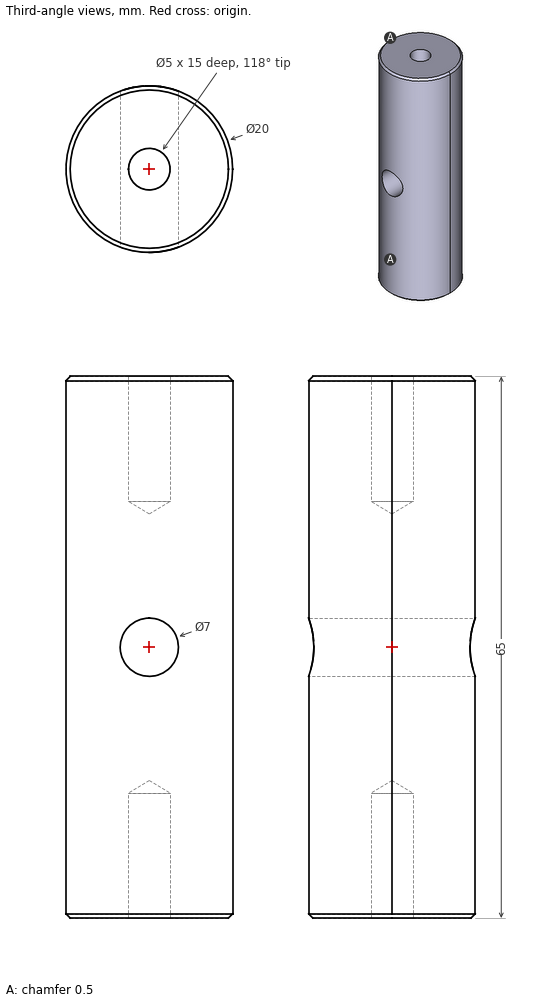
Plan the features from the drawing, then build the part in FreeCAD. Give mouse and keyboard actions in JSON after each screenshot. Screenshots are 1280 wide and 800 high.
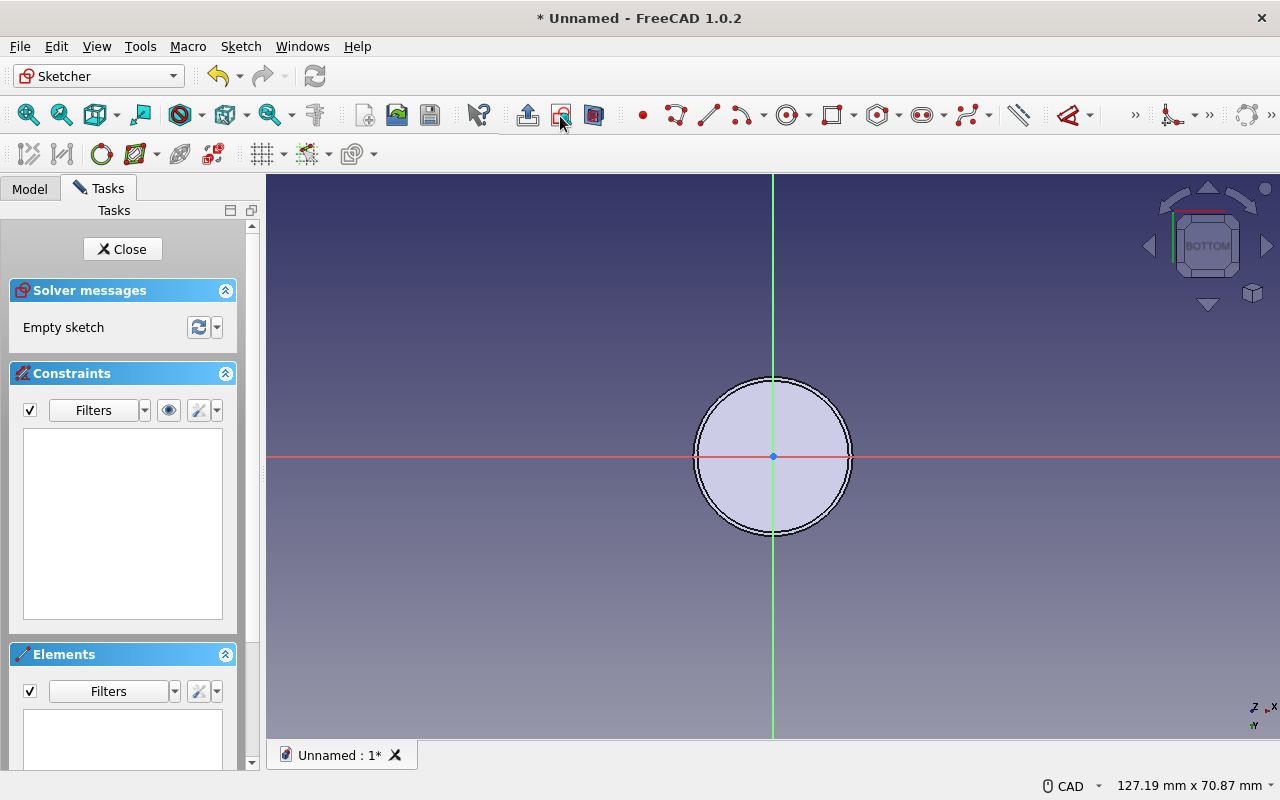
{"action": "scroll", "coordinate": [782, 456], "scroll_direction": "up", "scroll_amount": 11}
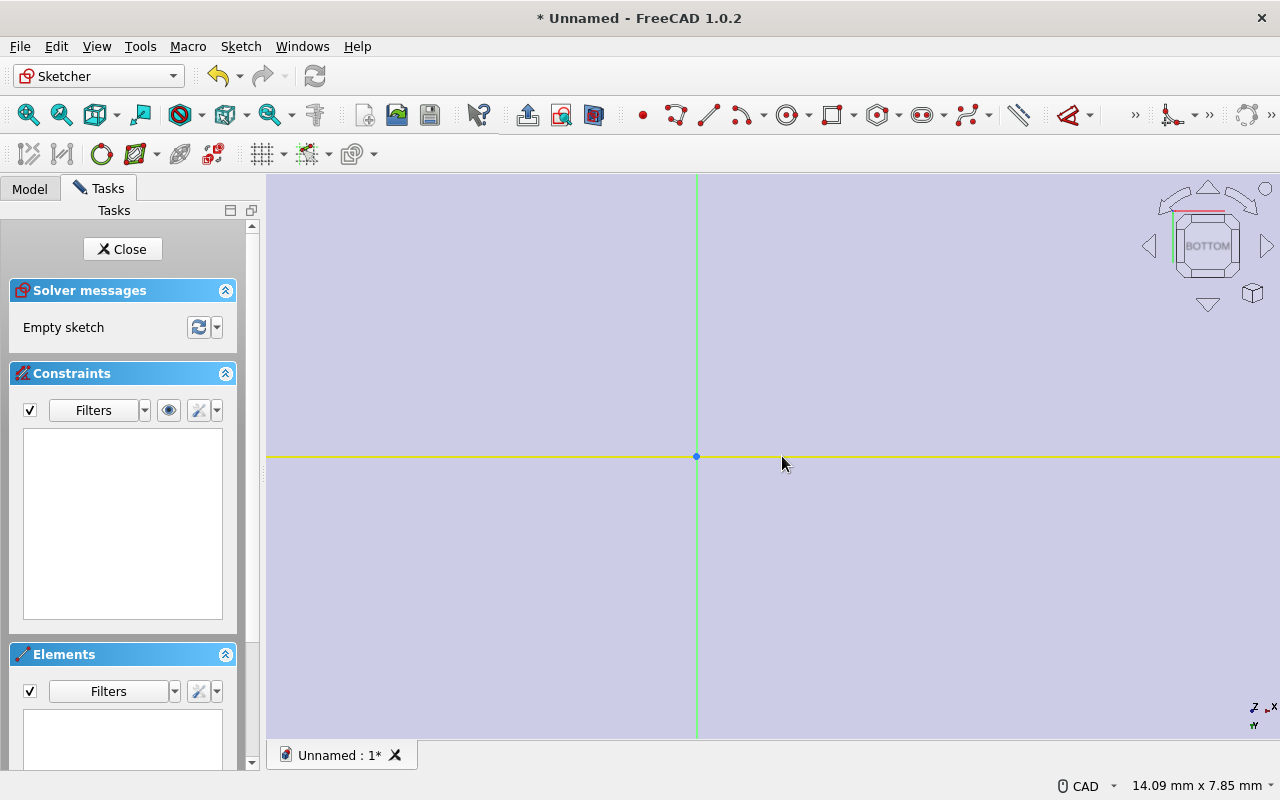
{"action": "left_click", "coordinate": [786, 116]}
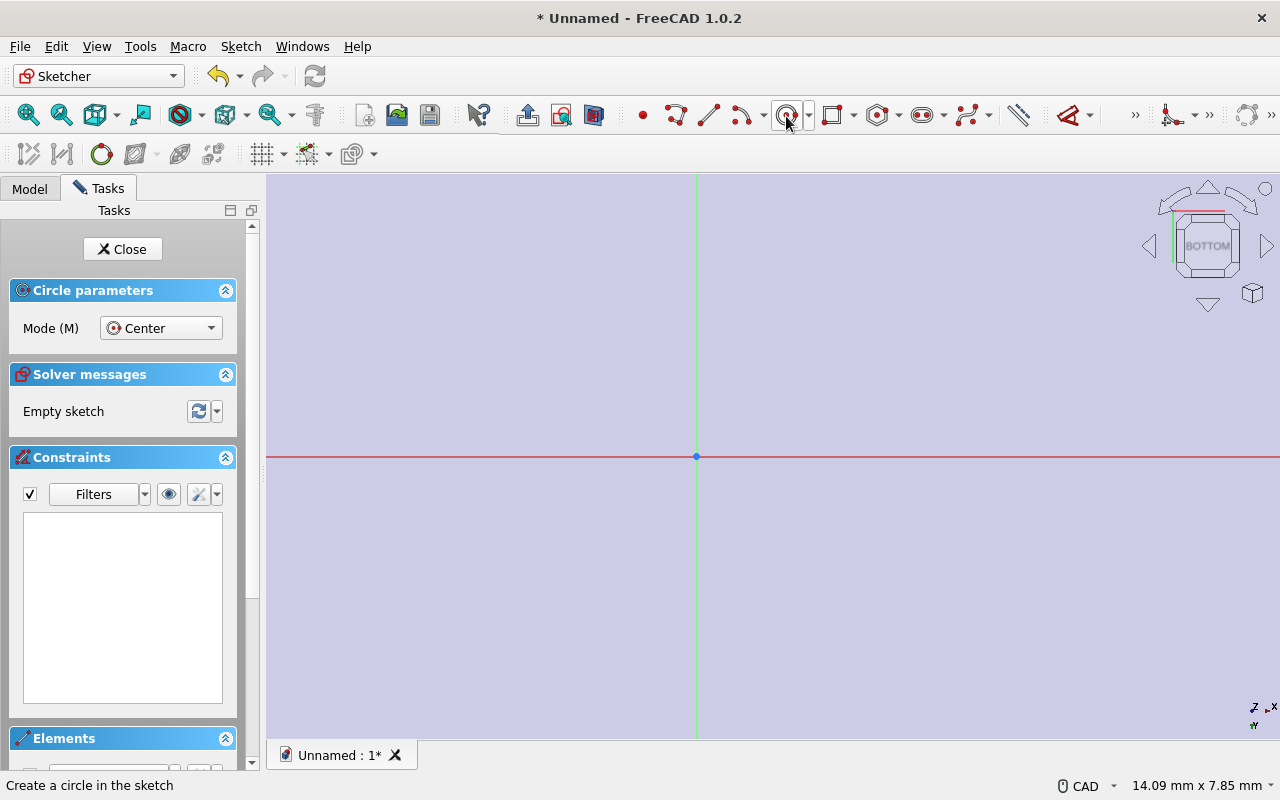
{"action": "left_click", "coordinate": [697, 456]}
{"action": "left_click", "coordinate": [824, 329]}
{"action": "key", "text": "Escape"}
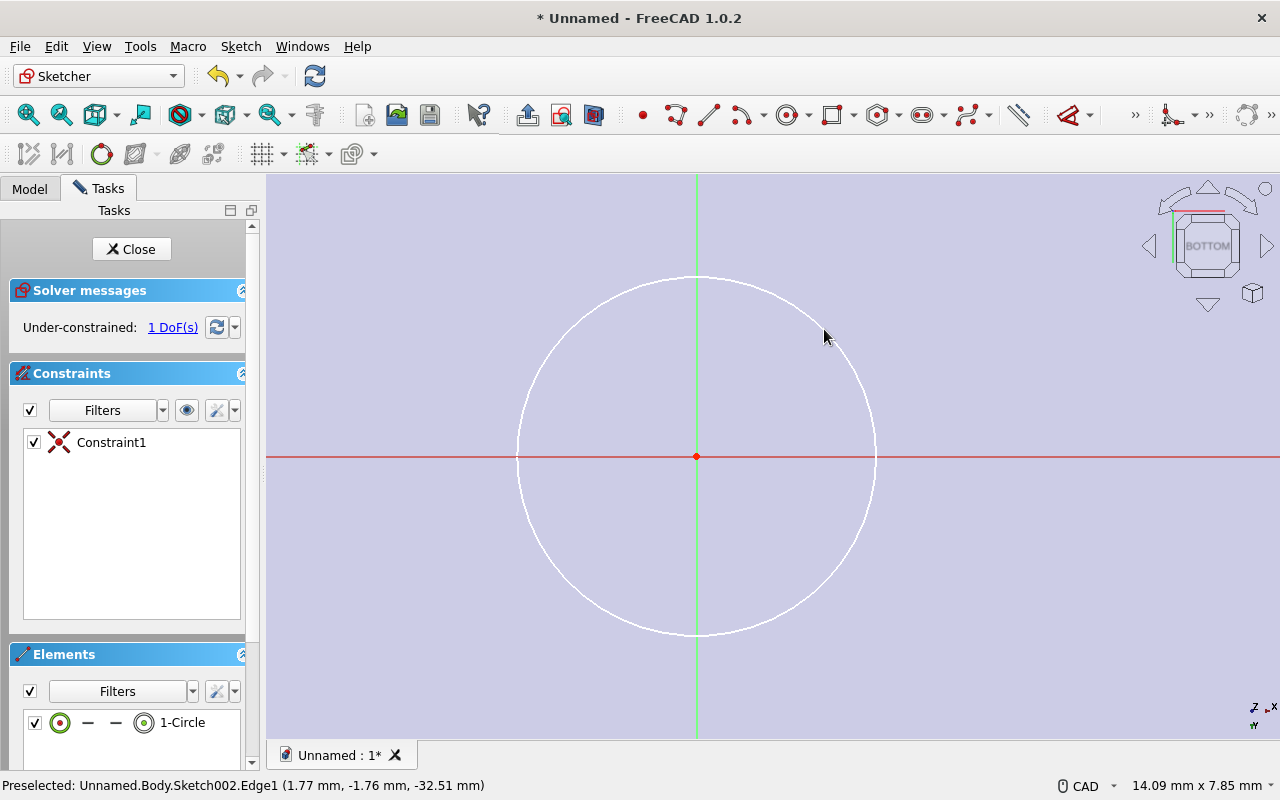
{"action": "left_click", "coordinate": [1068, 116]}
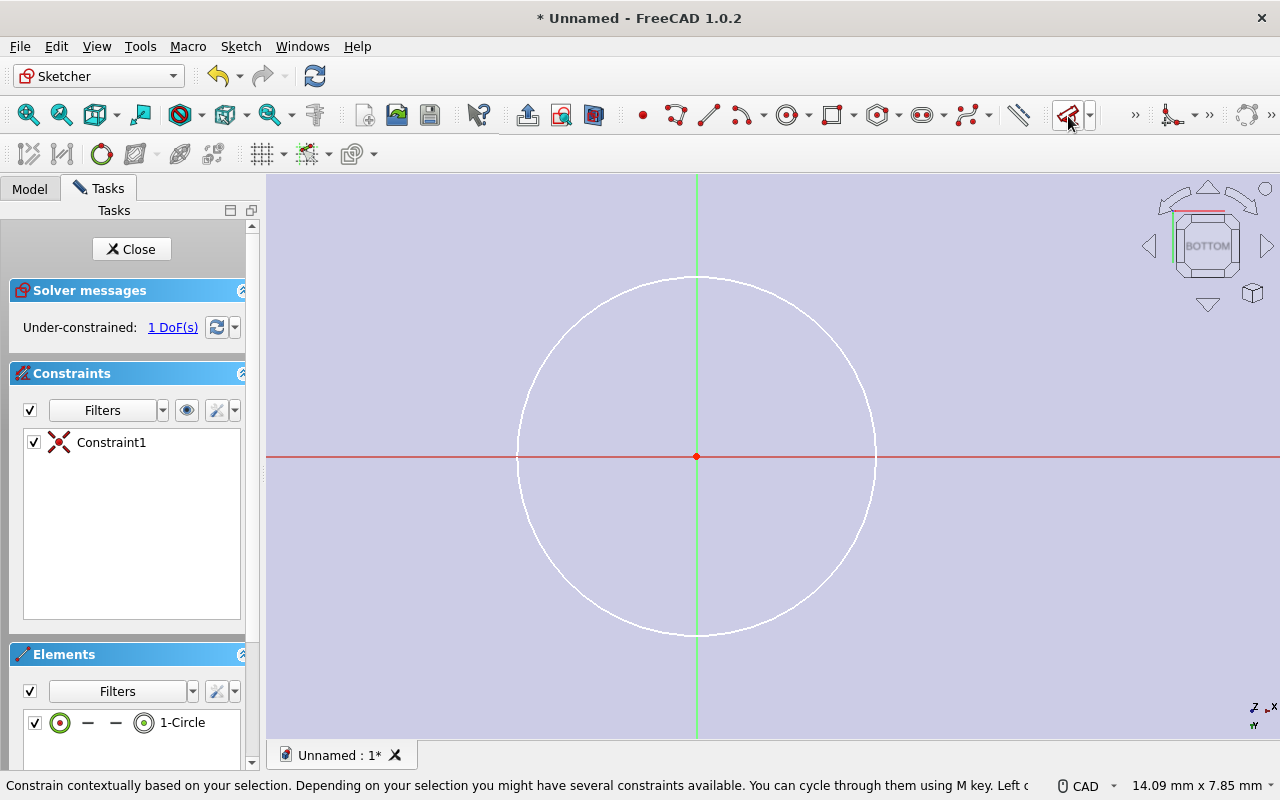
{"action": "left_click", "coordinate": [823, 329]}
{"action": "left_click", "coordinate": [846, 306]}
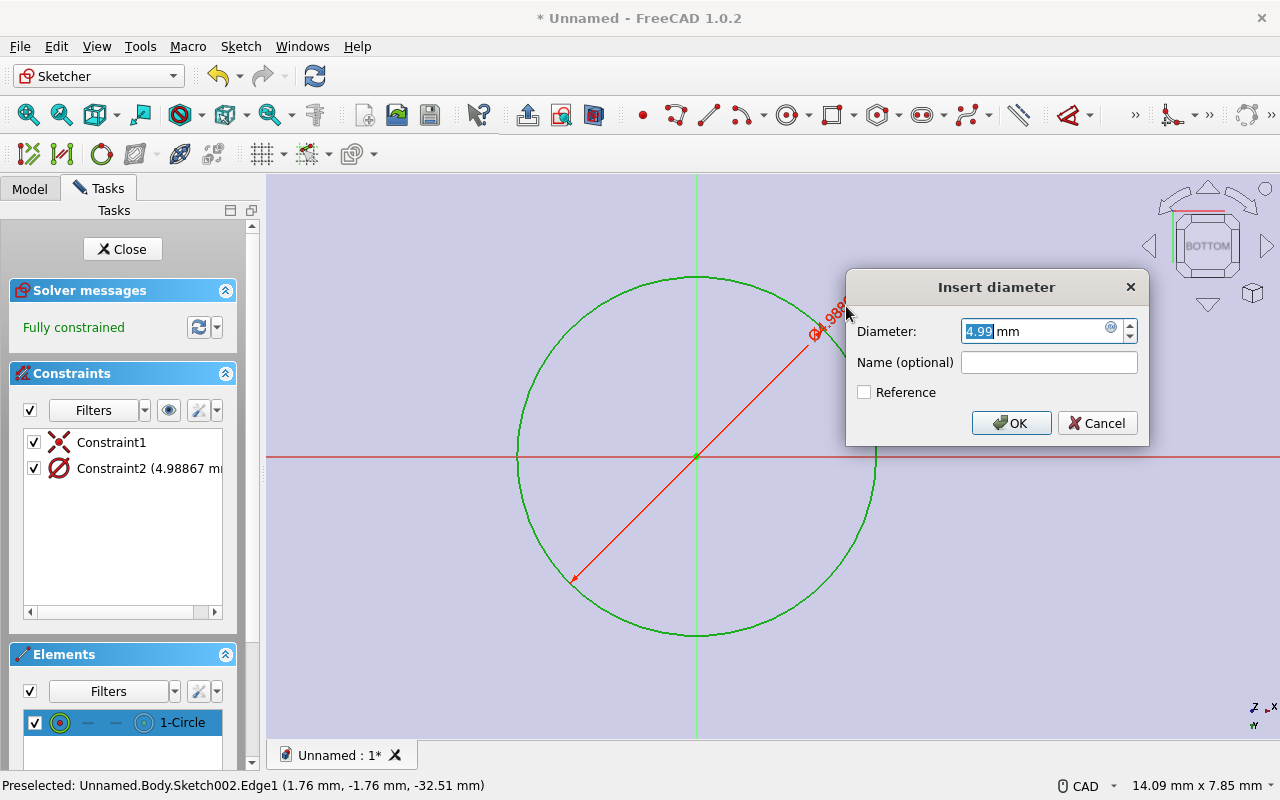
{"action": "type", "text": "5"}
{"action": "key", "text": "Return"}
{"action": "key", "text": "Escape"}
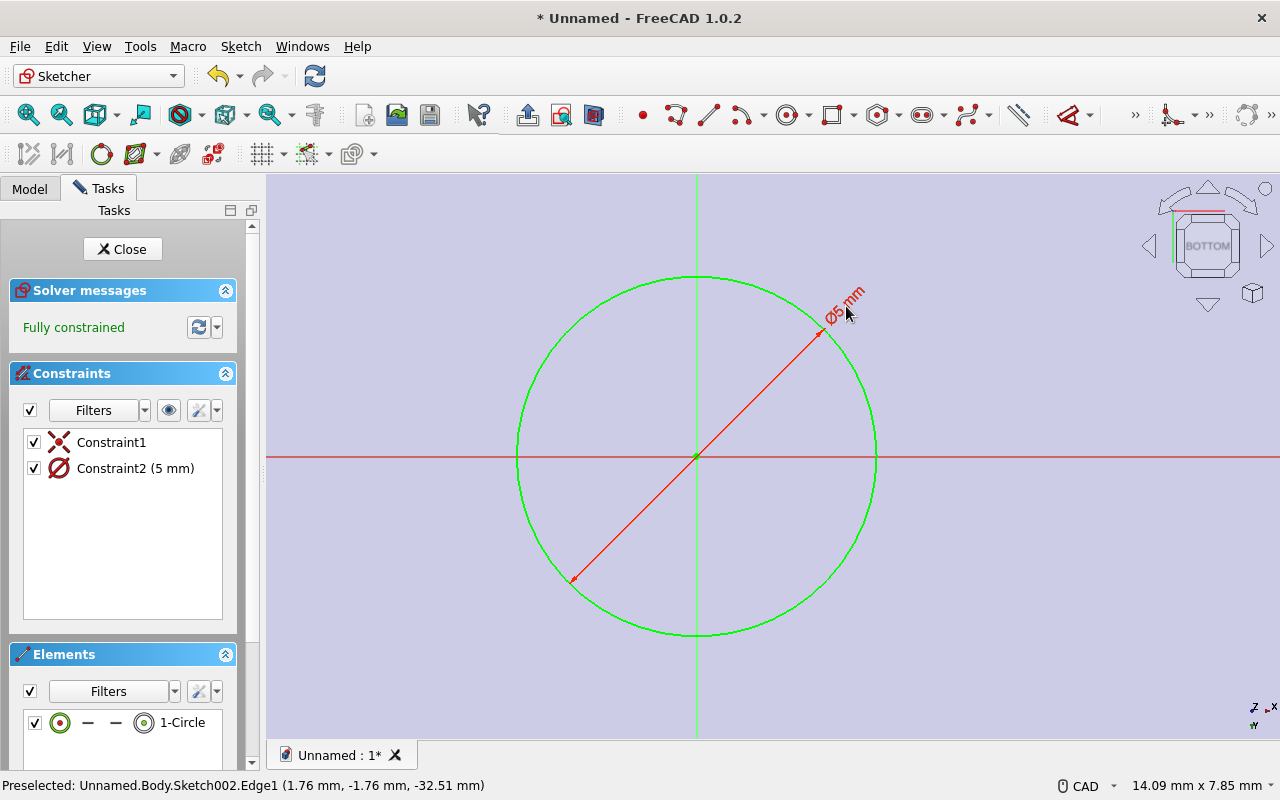
{"action": "left_click", "coordinate": [123, 249]}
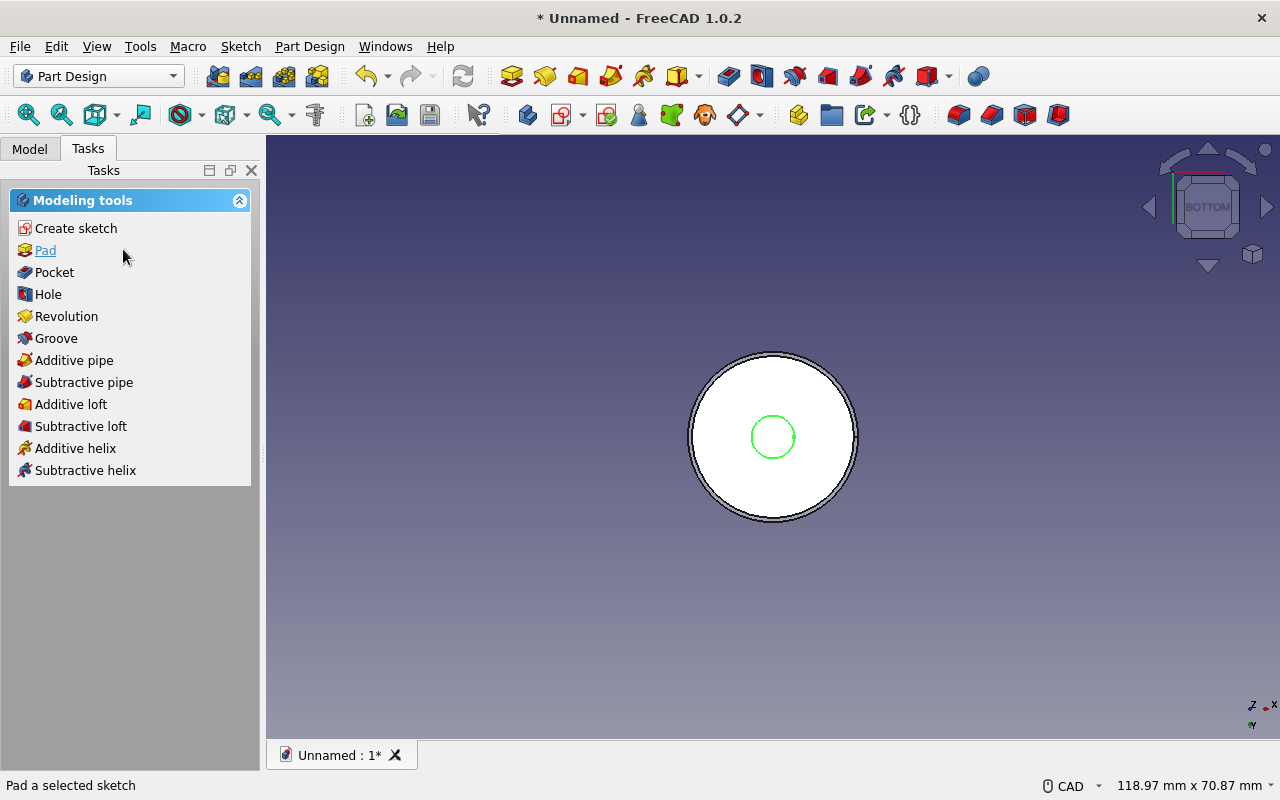
{"action": "left_click", "coordinate": [762, 76]}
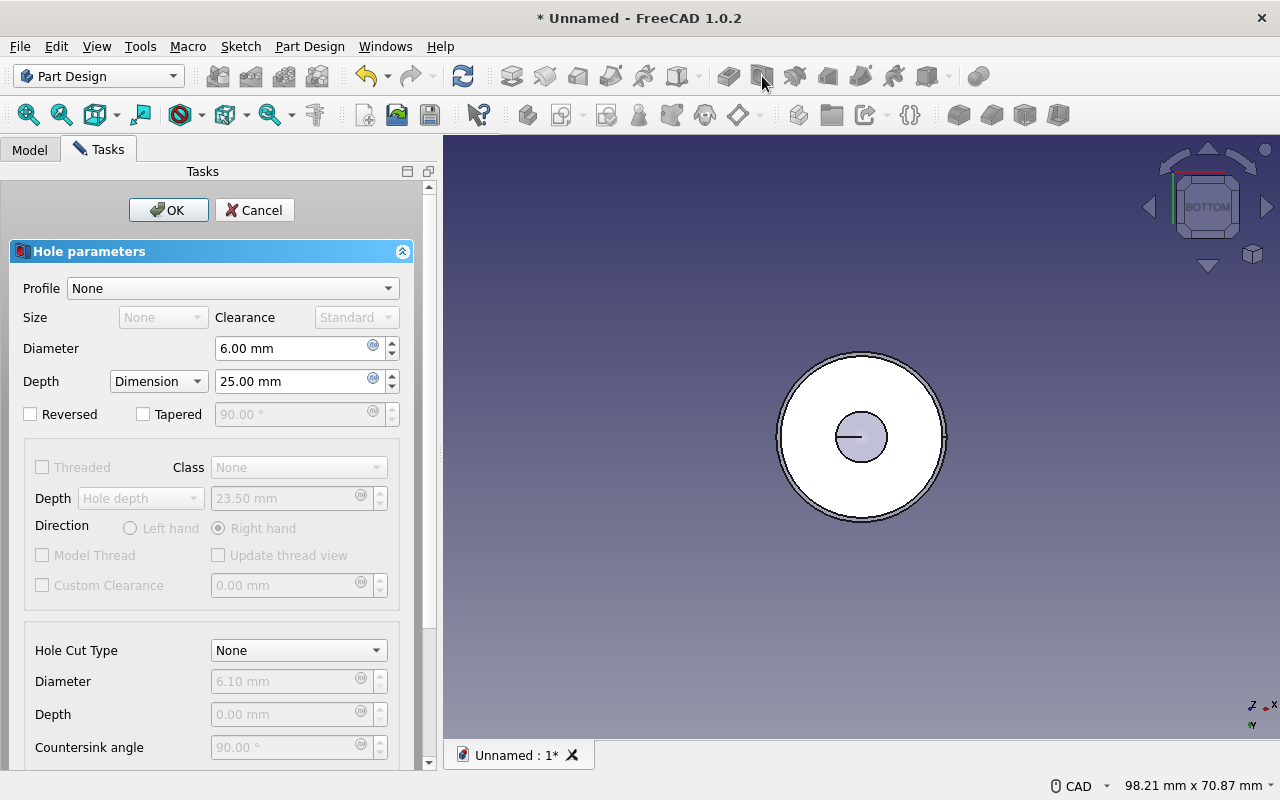
{"action": "triple_click", "coordinate": [300, 348]}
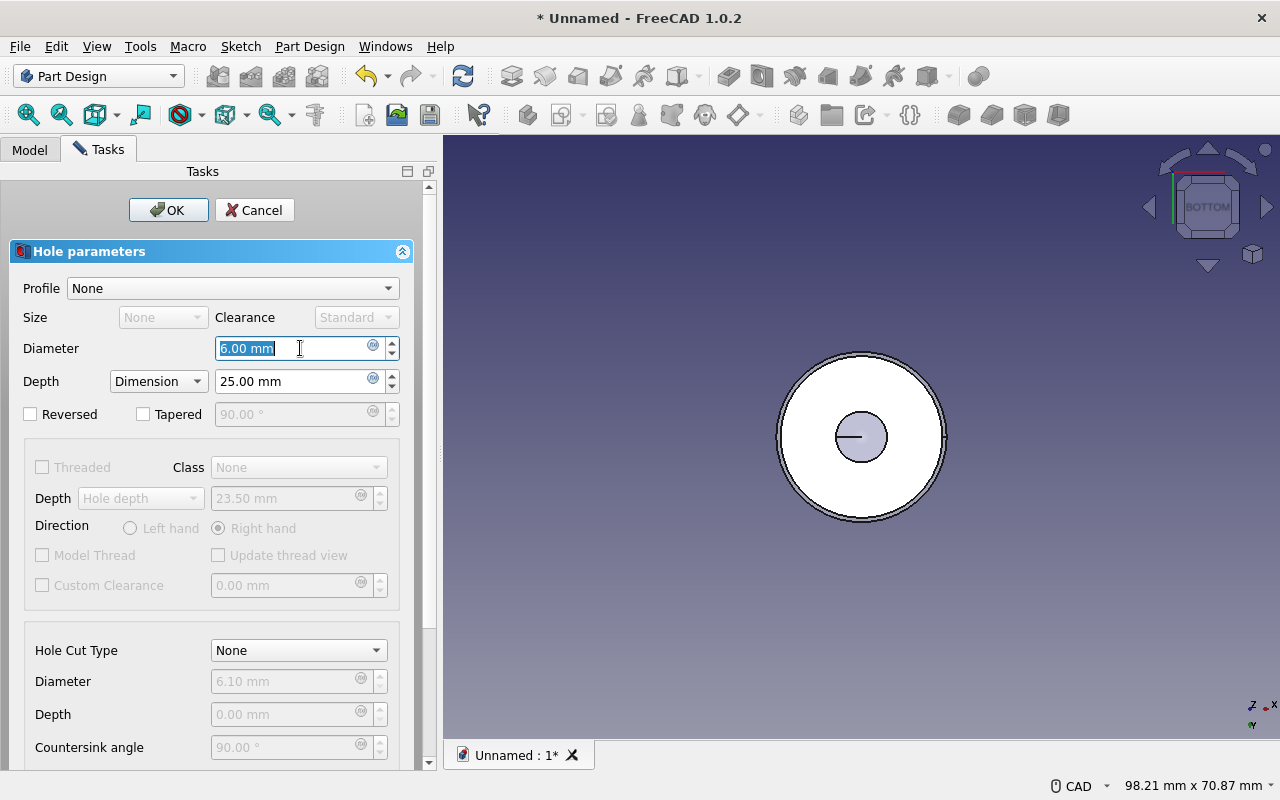
{"action": "type", "text": "5"}
{"action": "key", "text": "Tab"}